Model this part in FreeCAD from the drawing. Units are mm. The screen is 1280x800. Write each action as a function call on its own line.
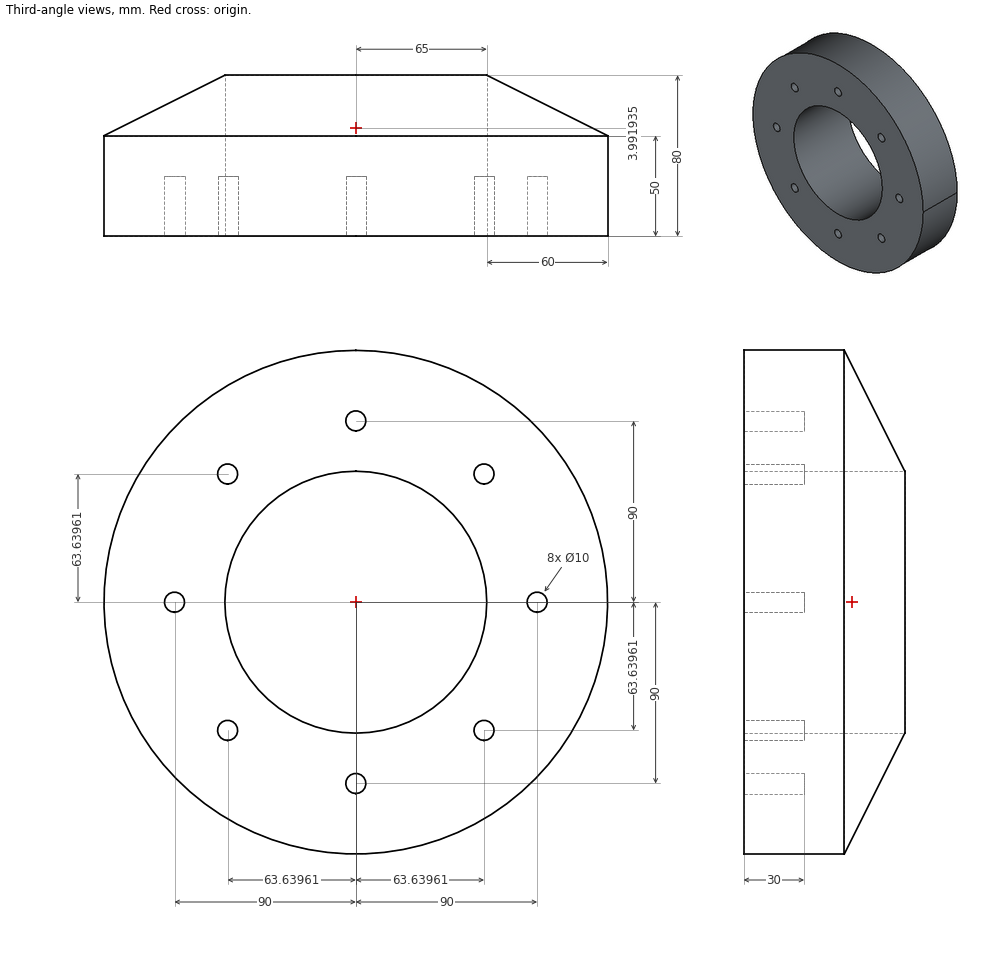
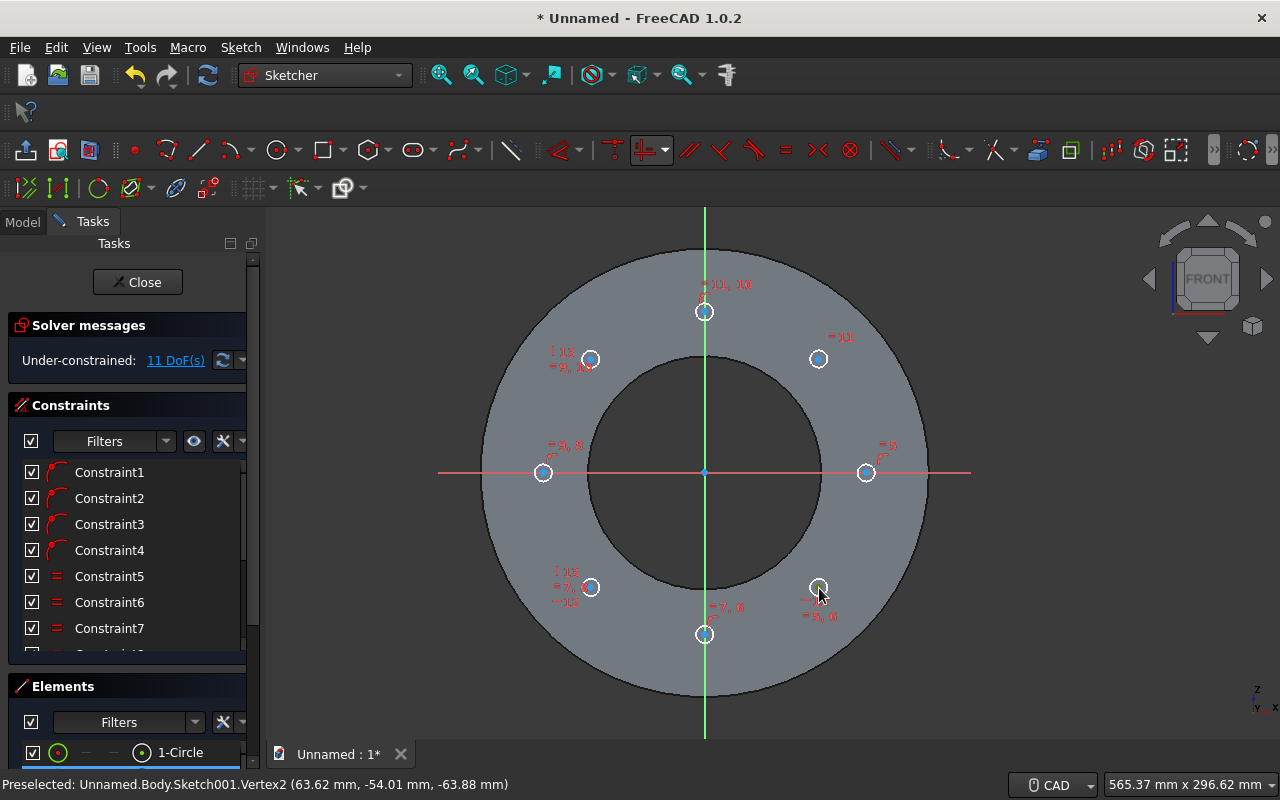
click(819, 359)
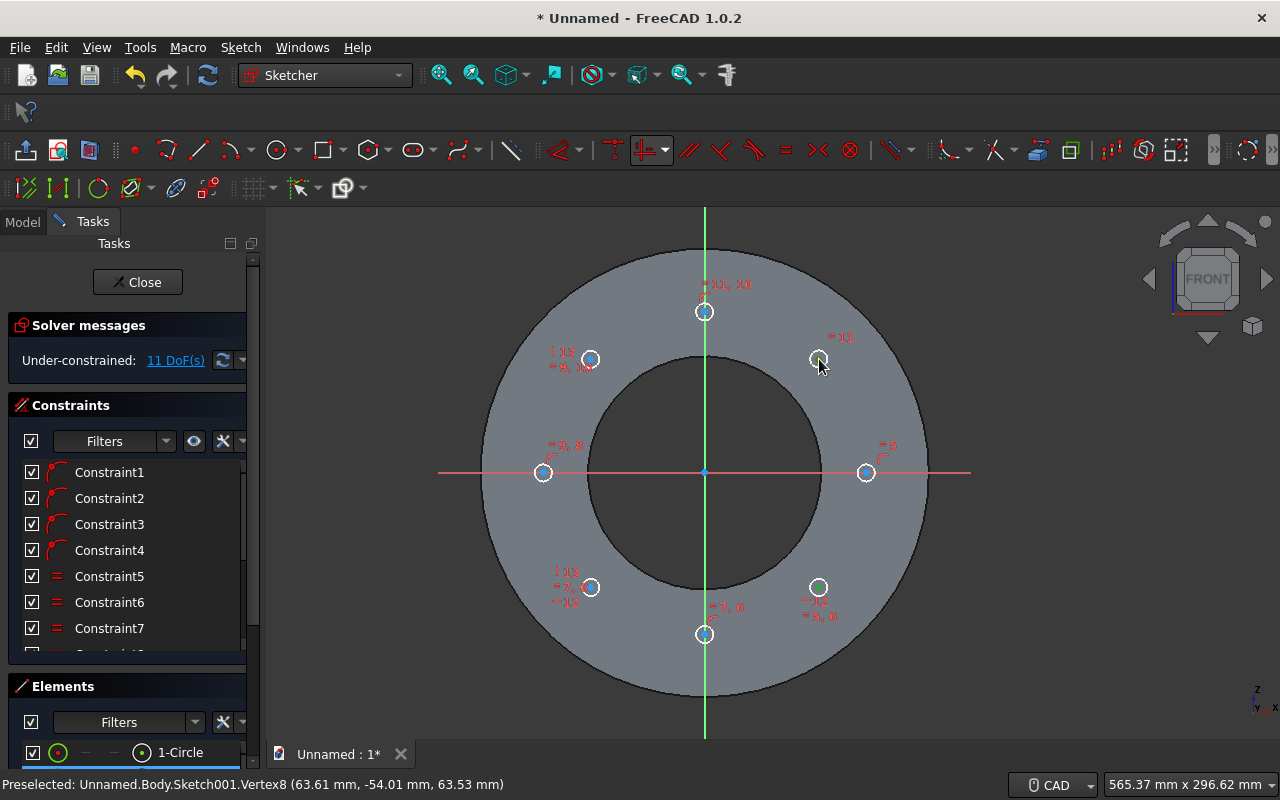
key(v)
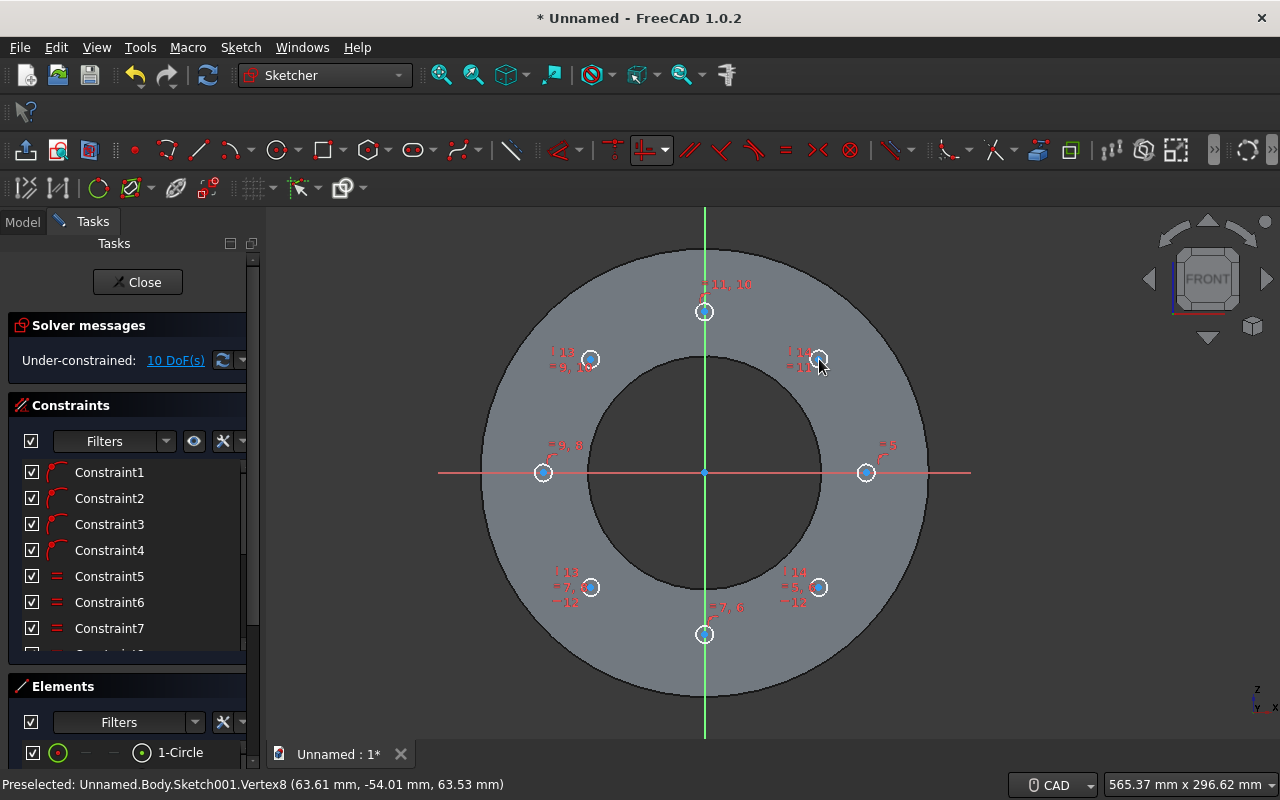
click(593, 361)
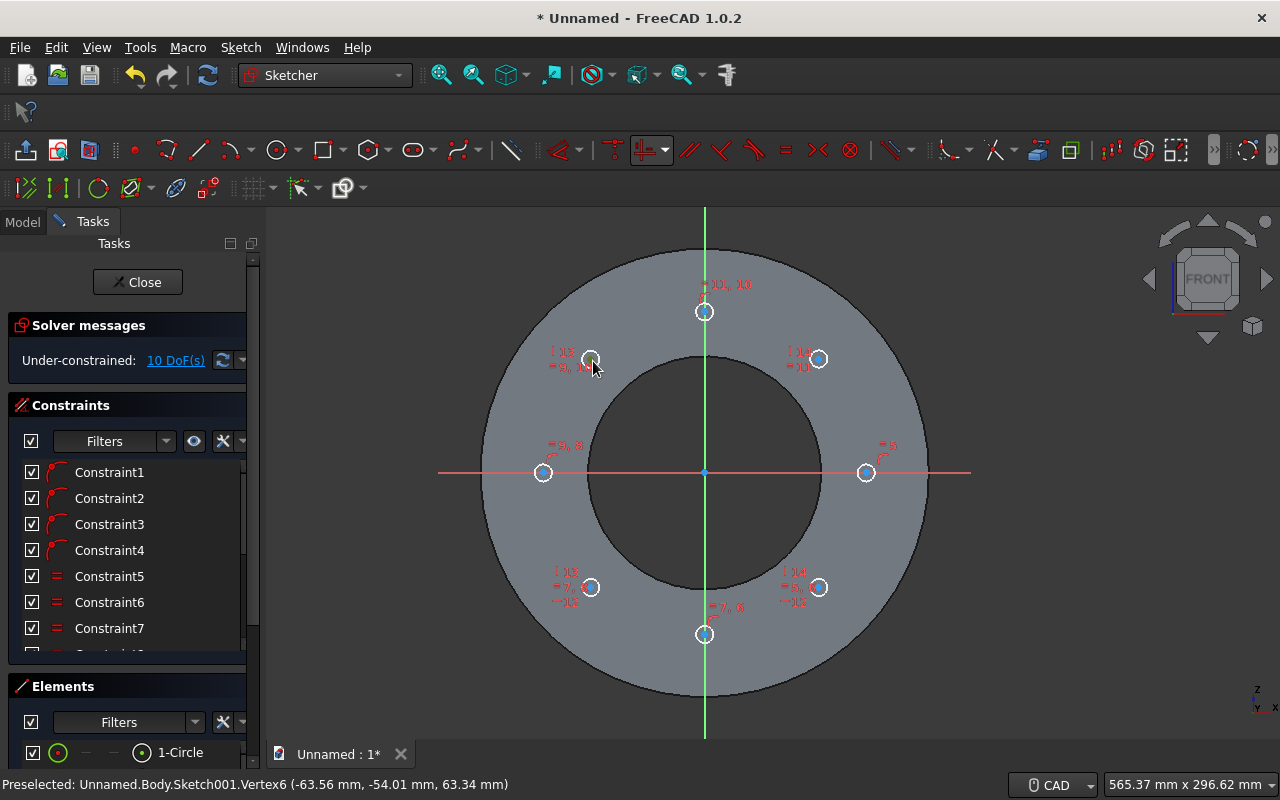
click(819, 359)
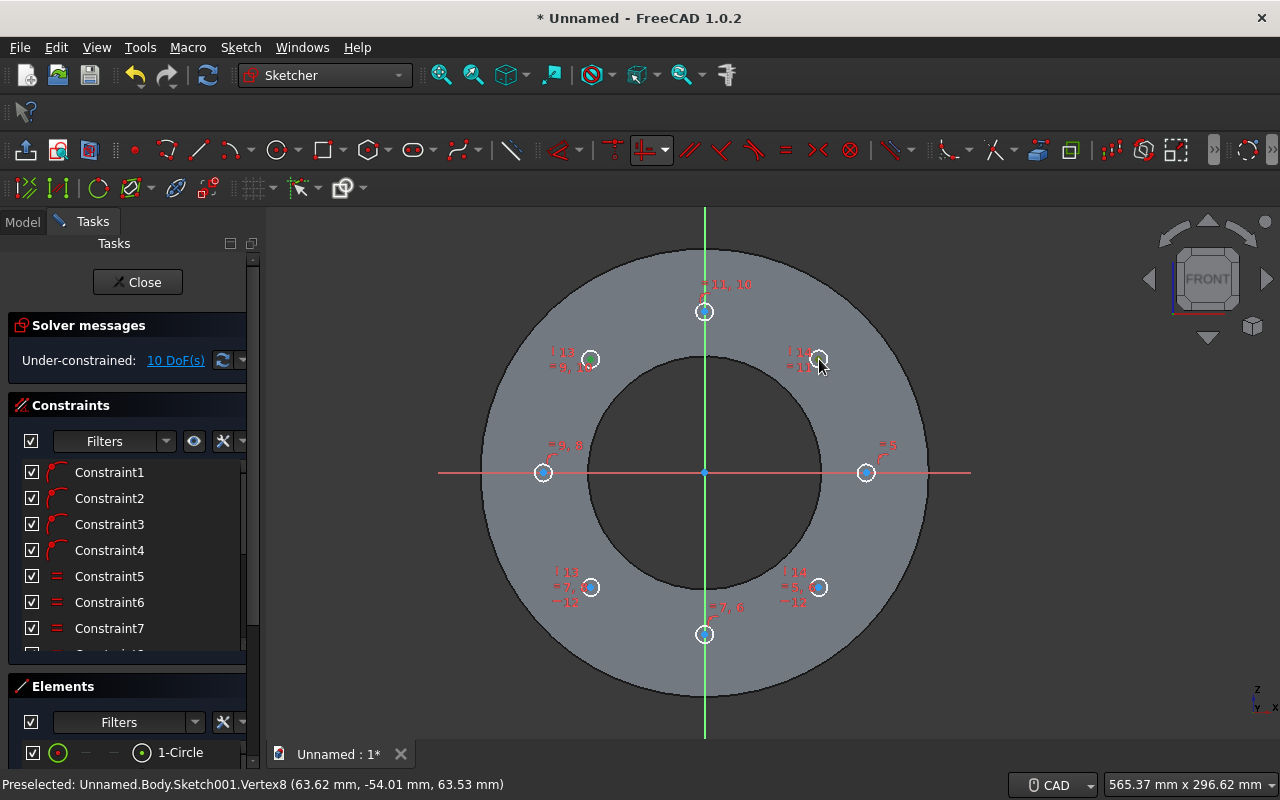
key(h)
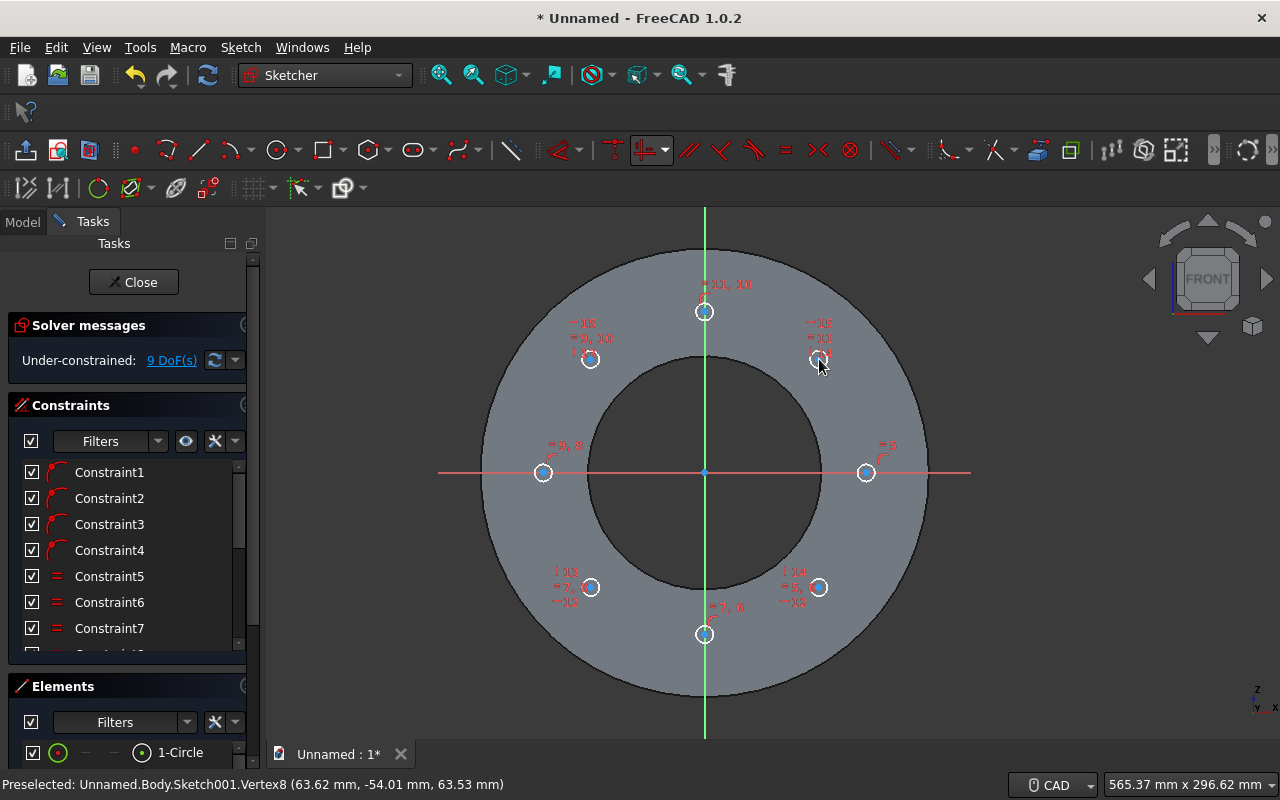
click(558, 150)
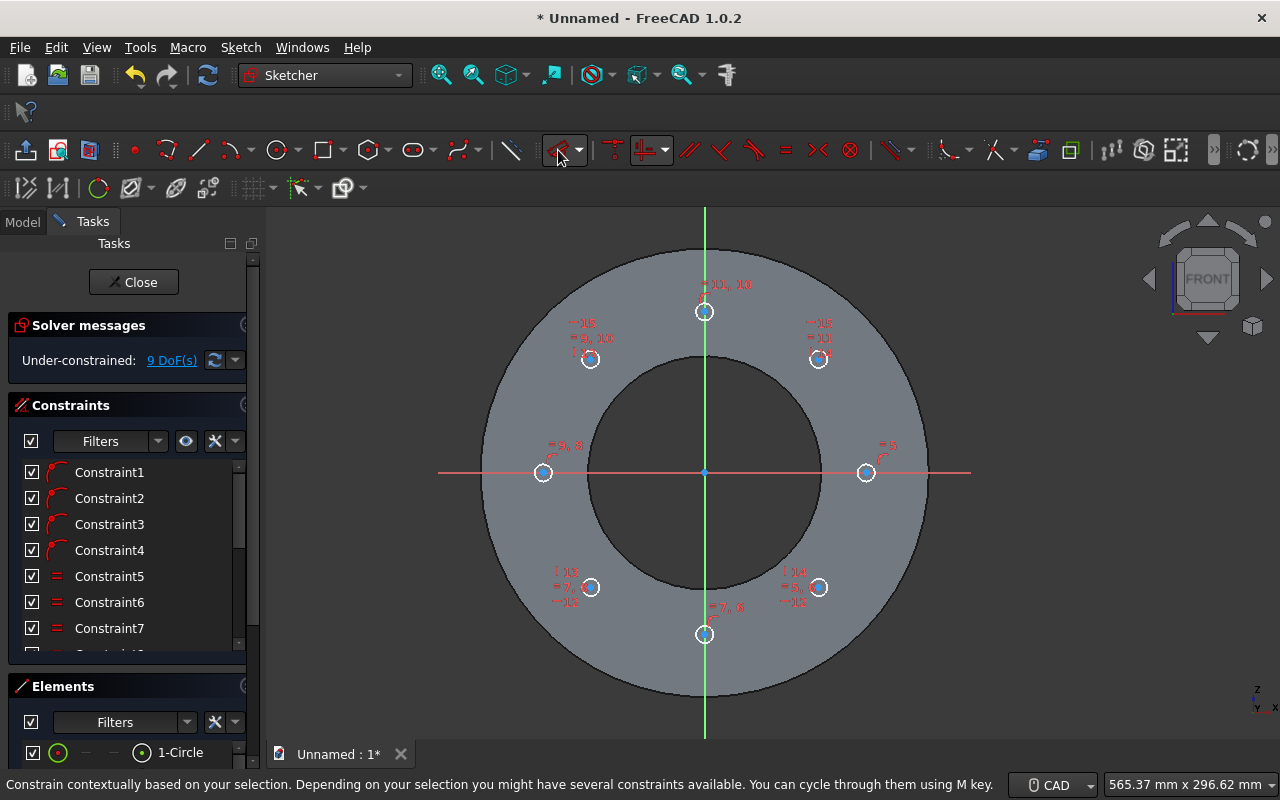
scroll(858, 473, up, 4)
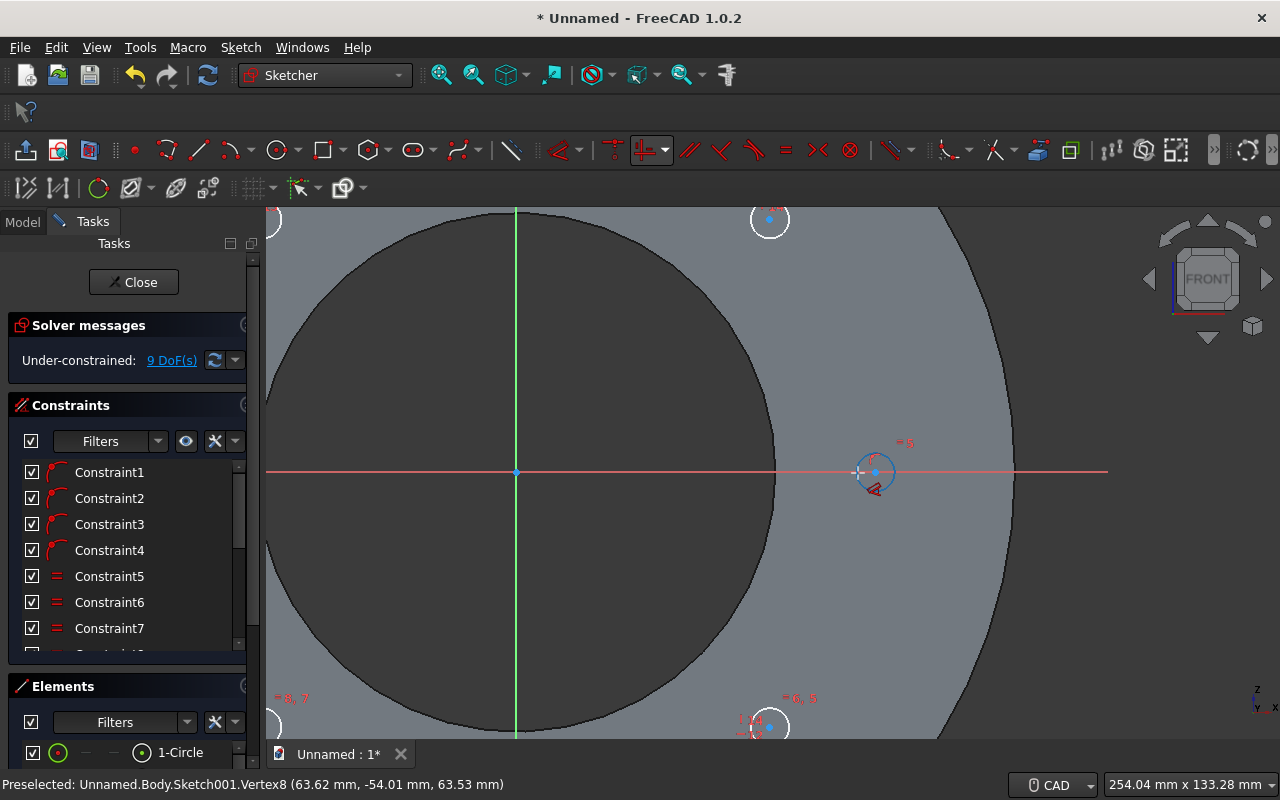
click(857, 472)
click(832, 447)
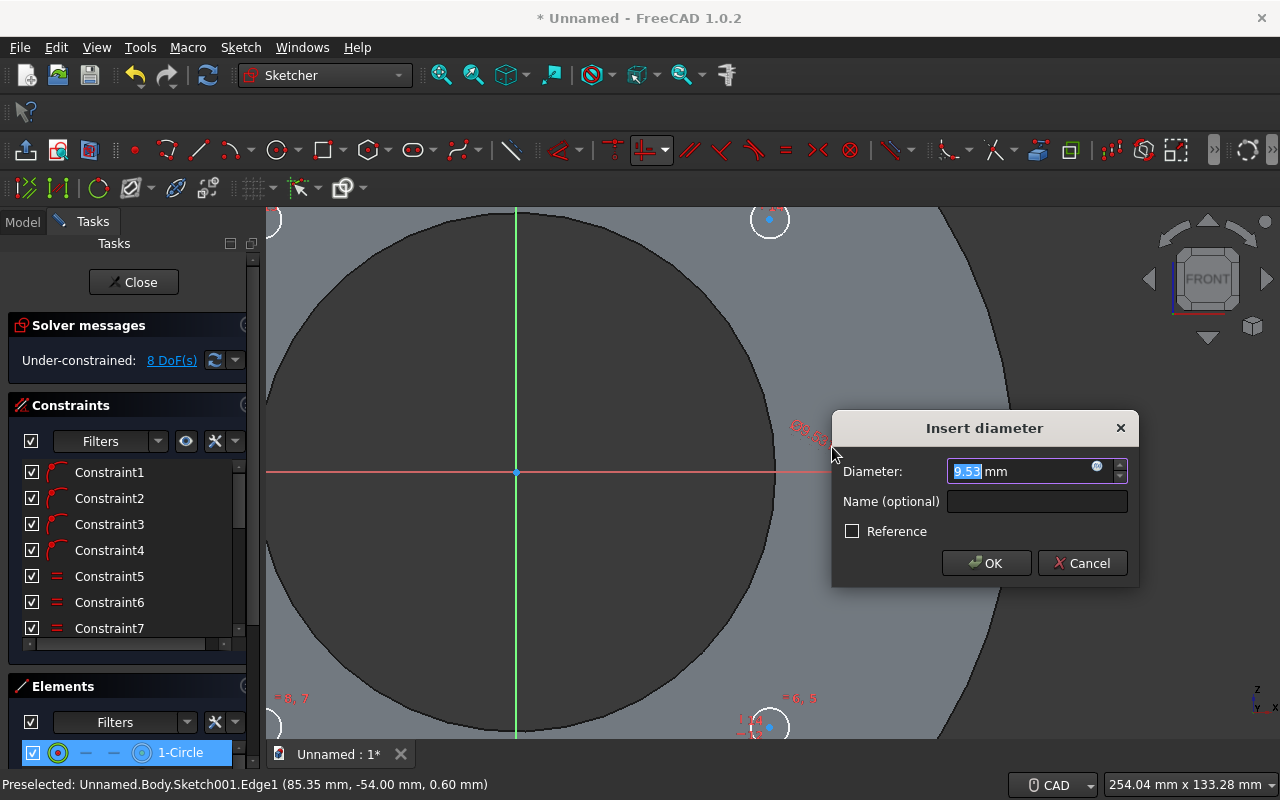
text(10)
key(Return)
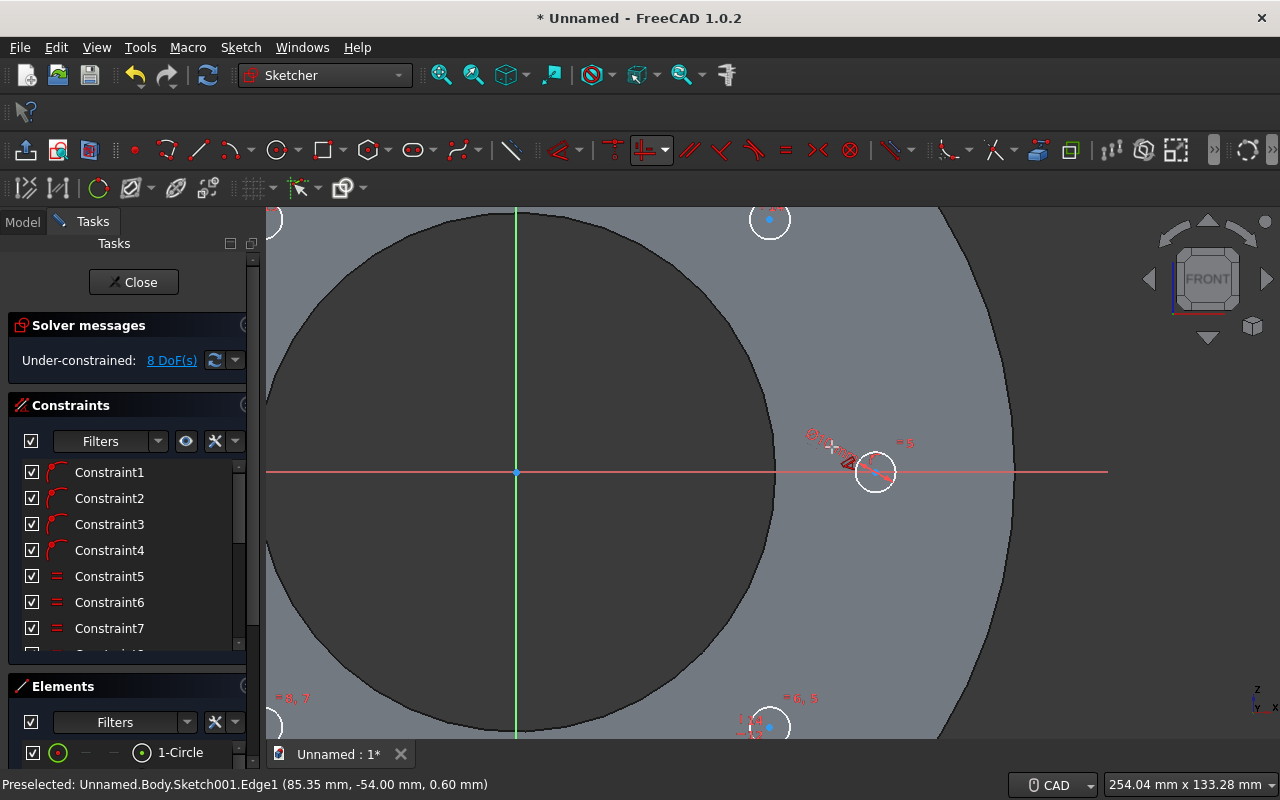
click(876, 472)
click(696, 506)